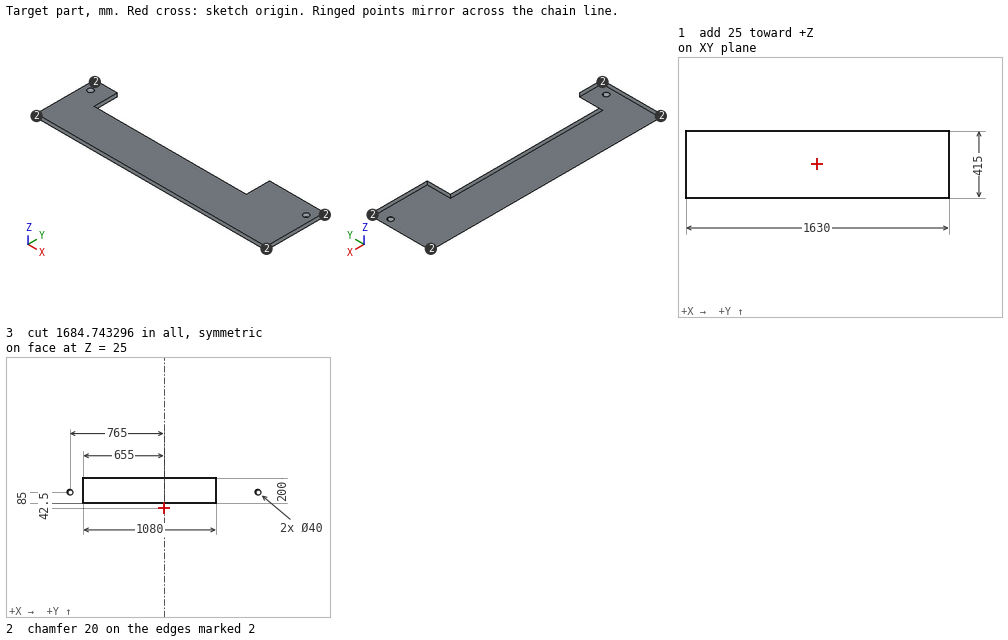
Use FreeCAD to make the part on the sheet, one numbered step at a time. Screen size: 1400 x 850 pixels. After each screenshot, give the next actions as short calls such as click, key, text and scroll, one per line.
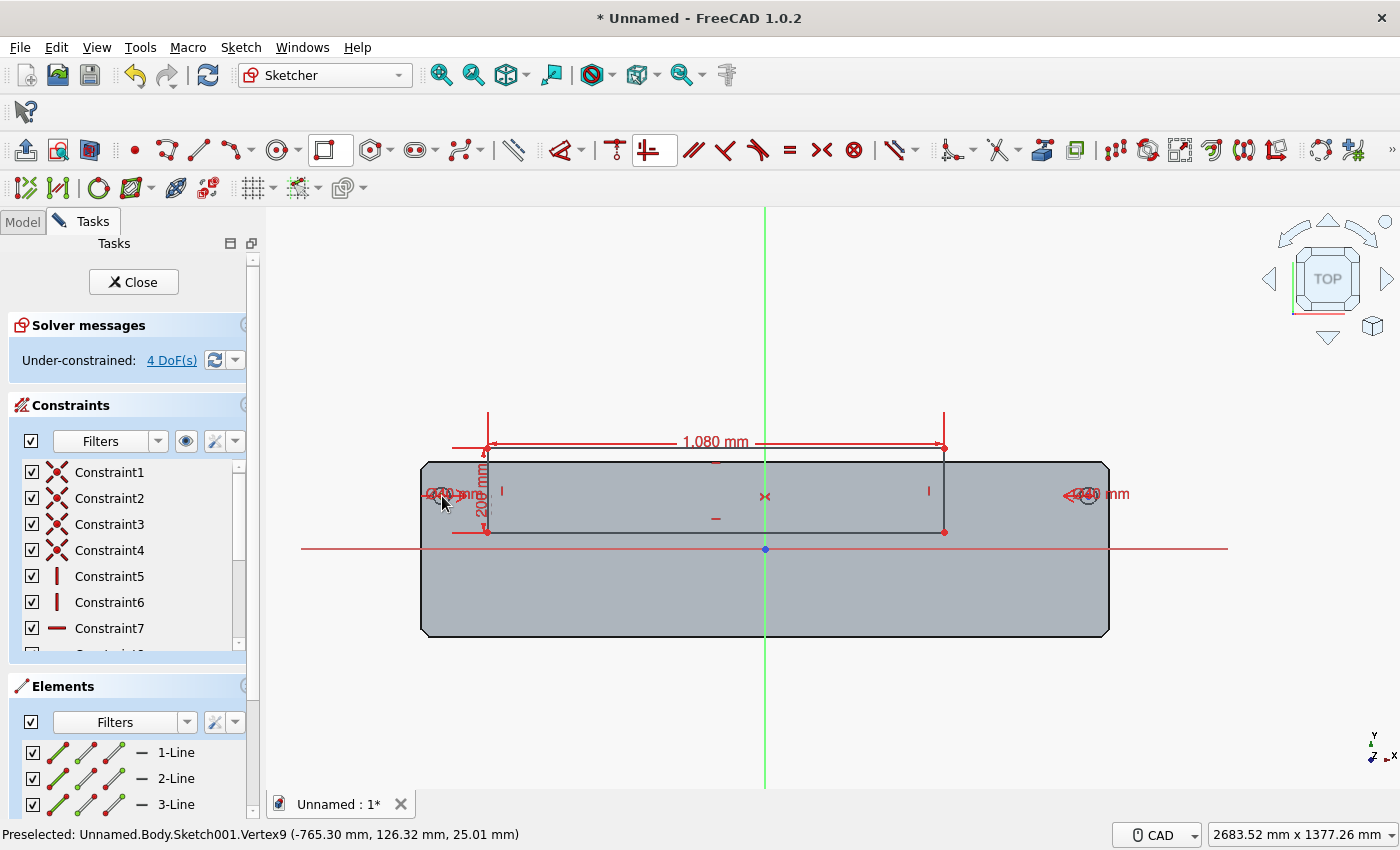
key(l)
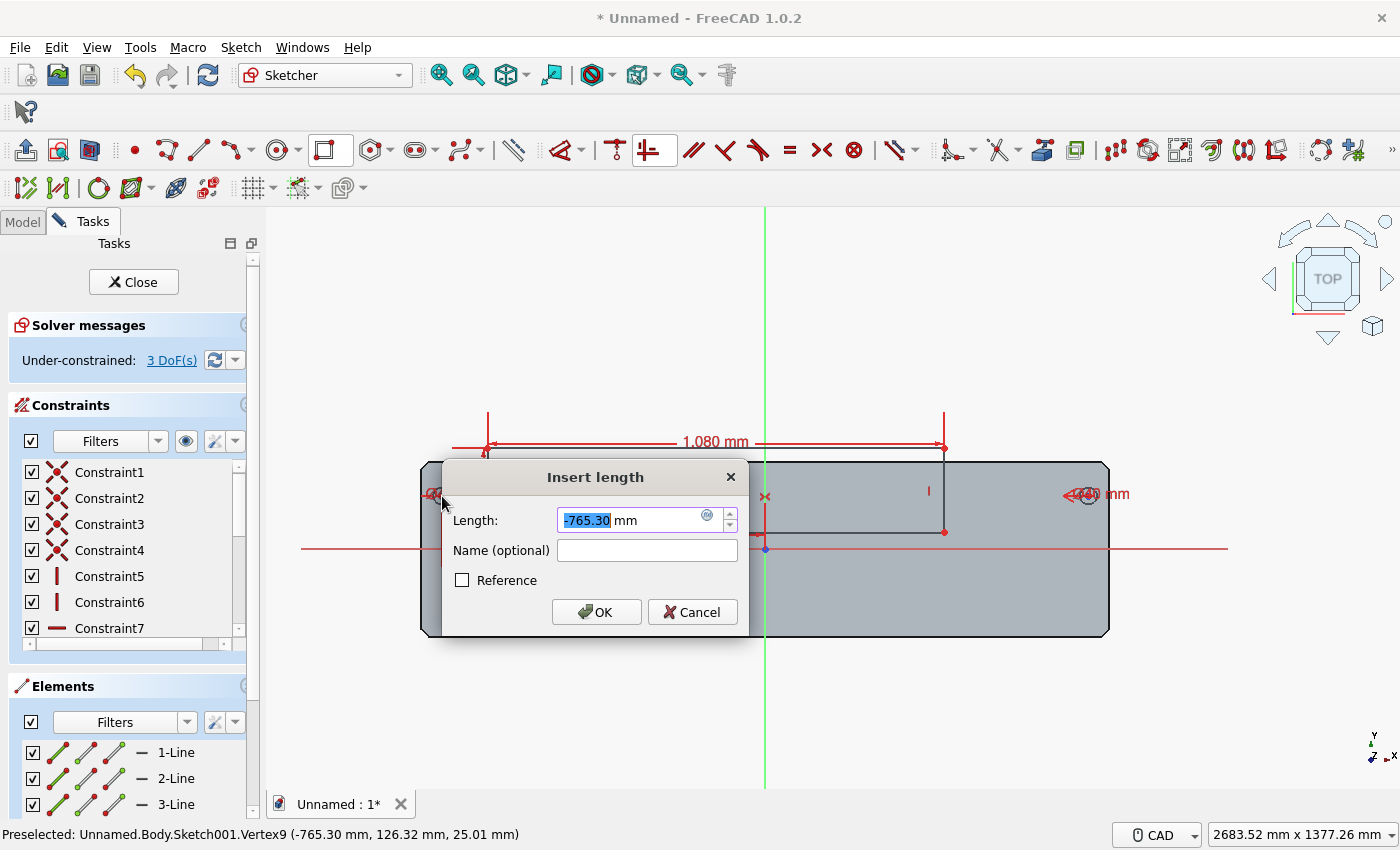
text(-765)
key(Return)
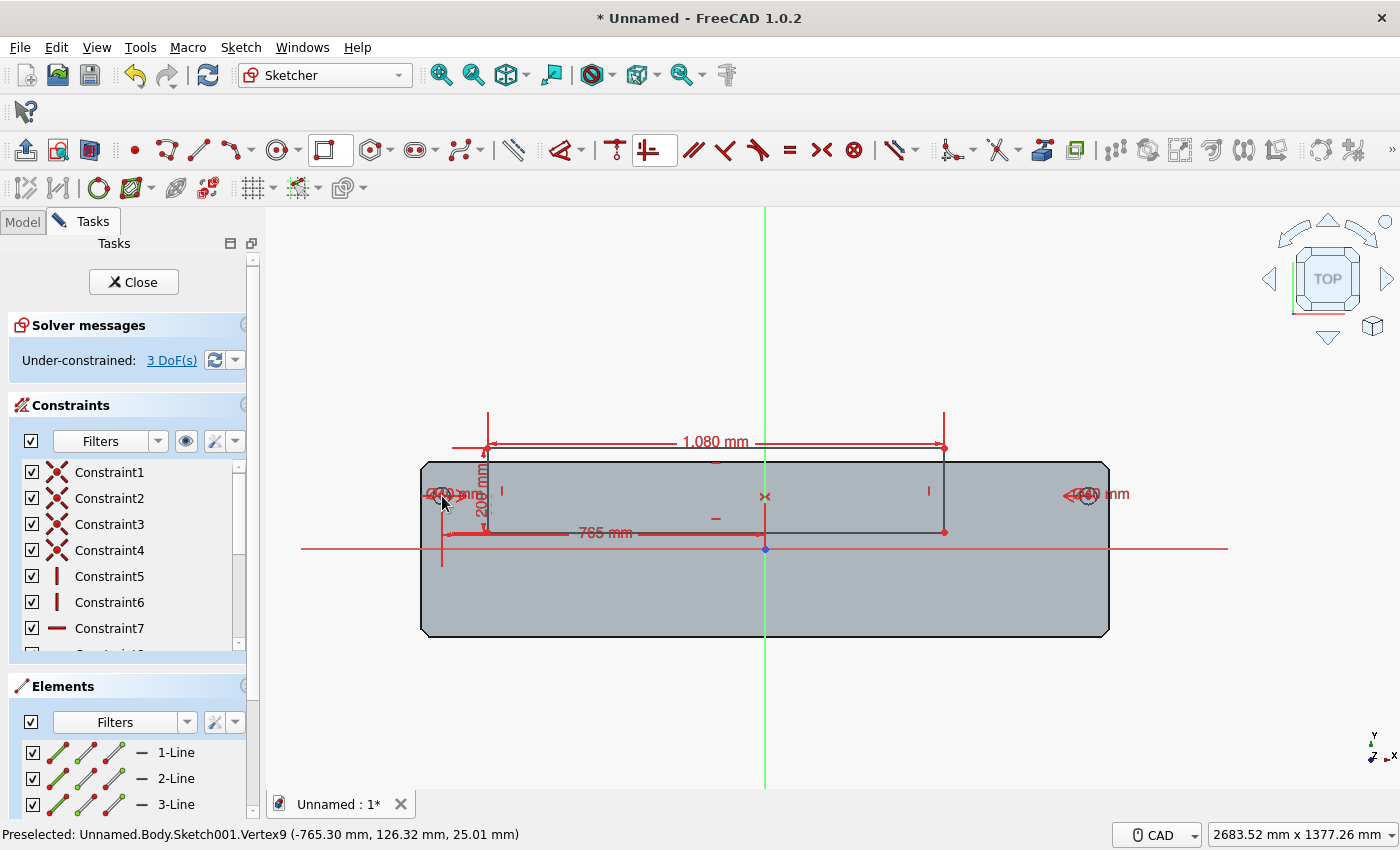
click(488, 533)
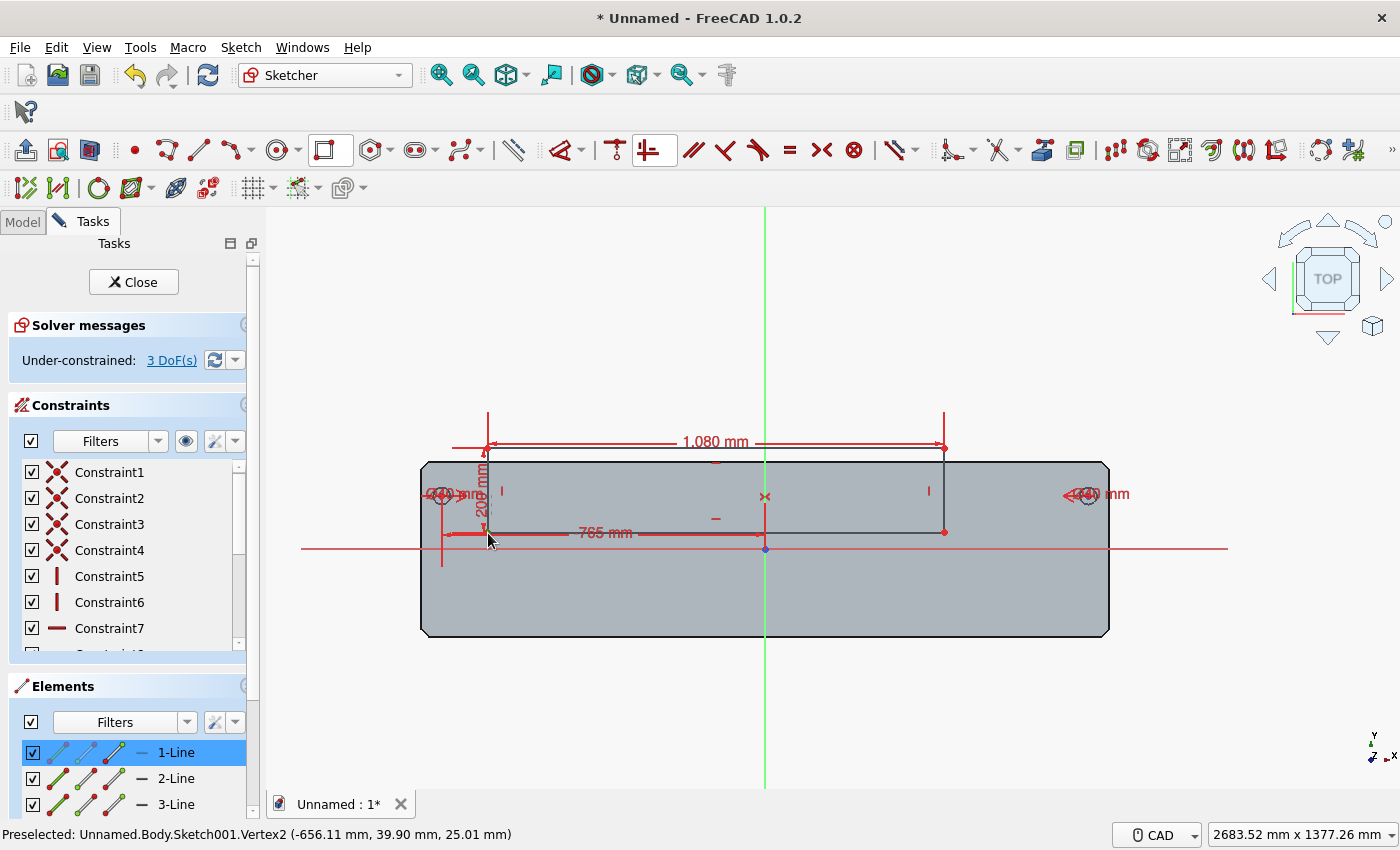
click(442, 496)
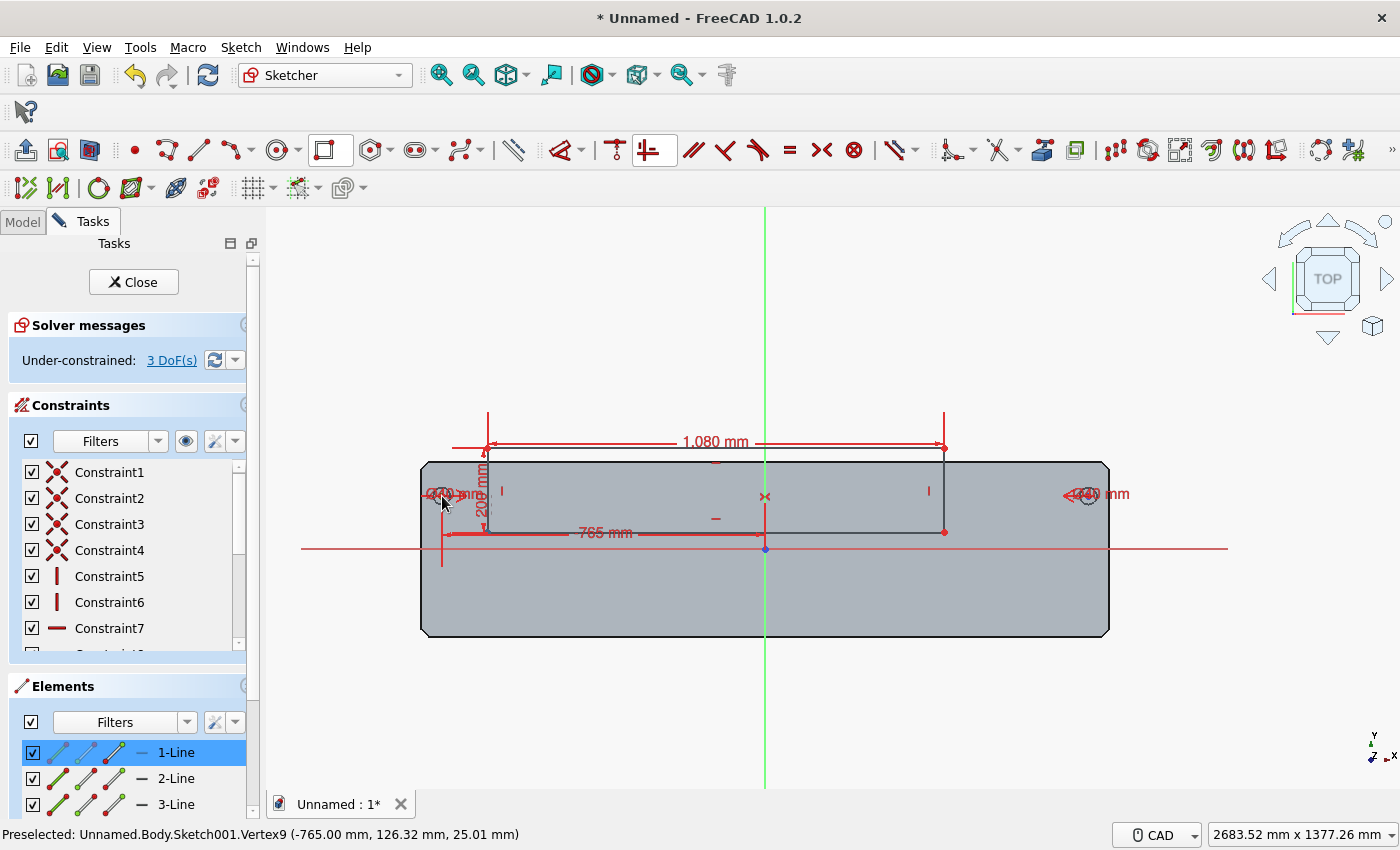
key(i)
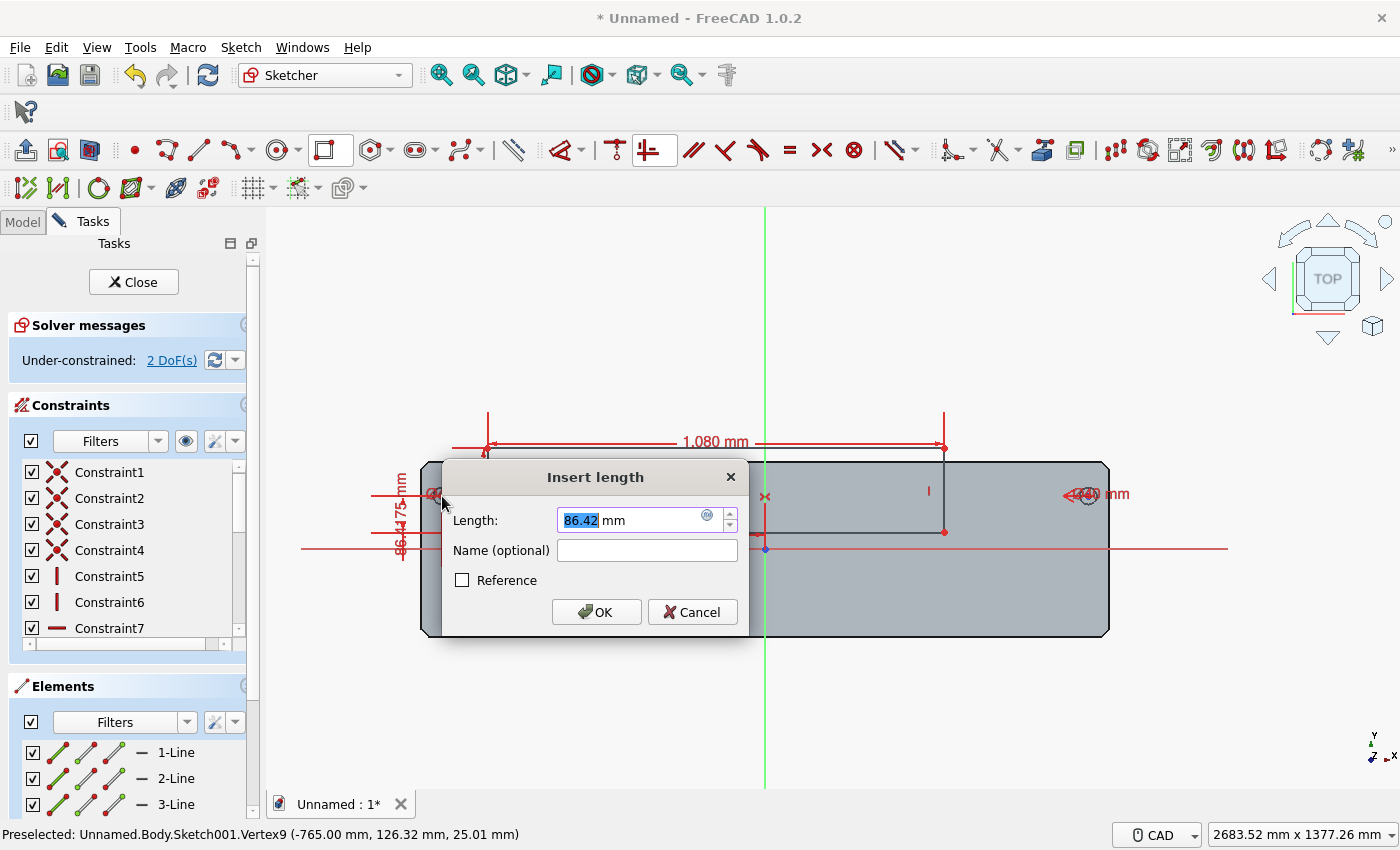
text(85)
key(Return)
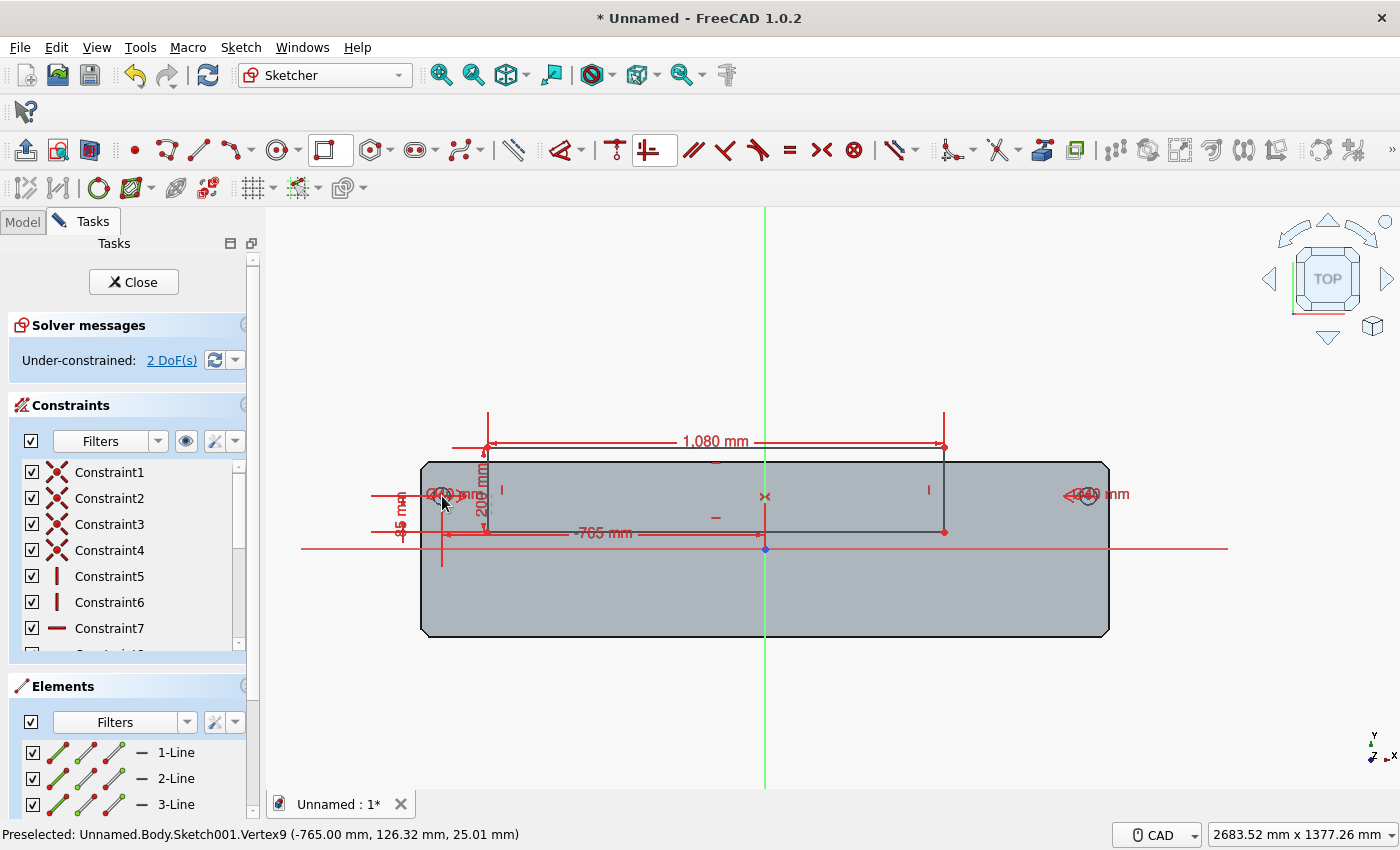
click(488, 448)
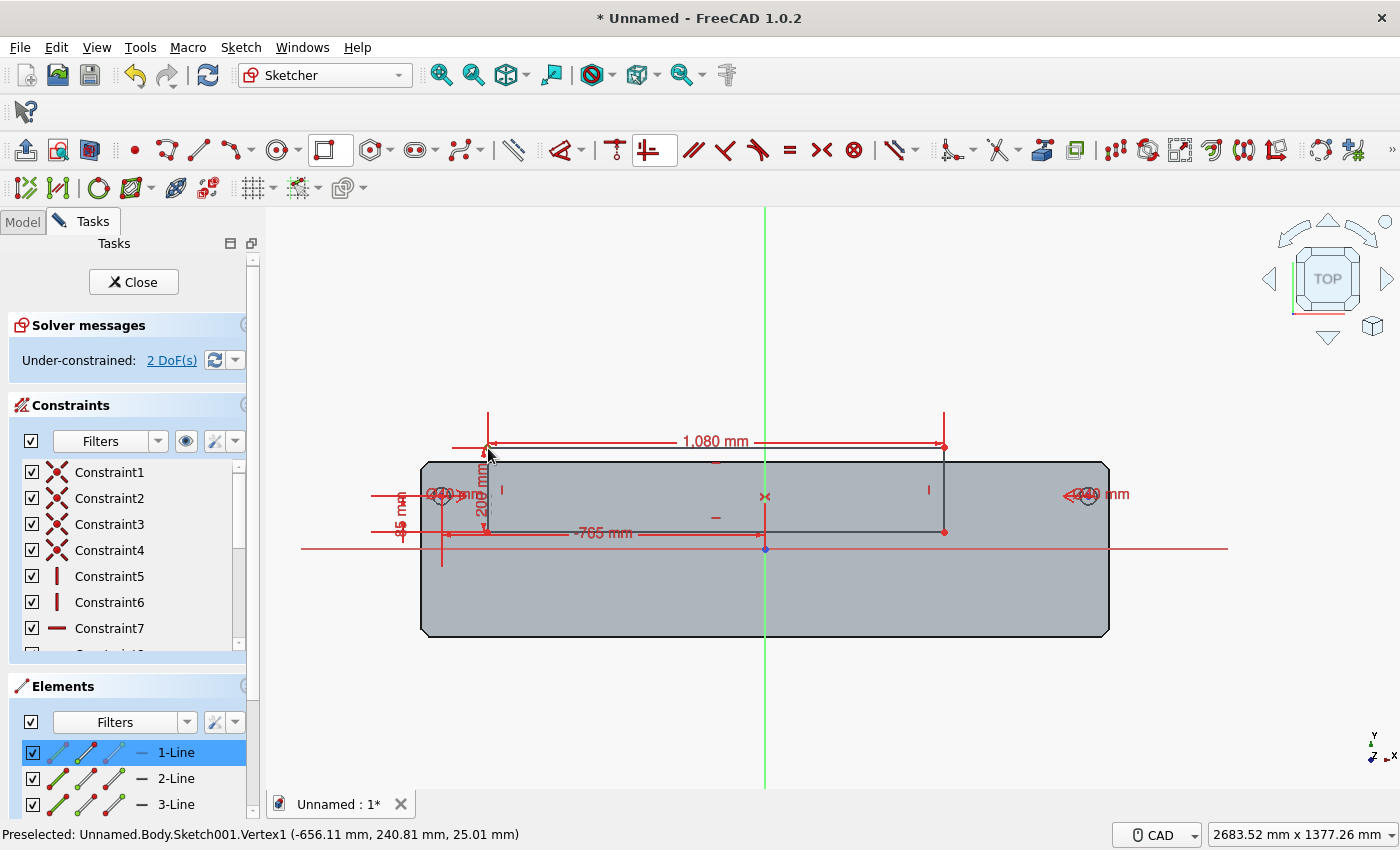
key(l)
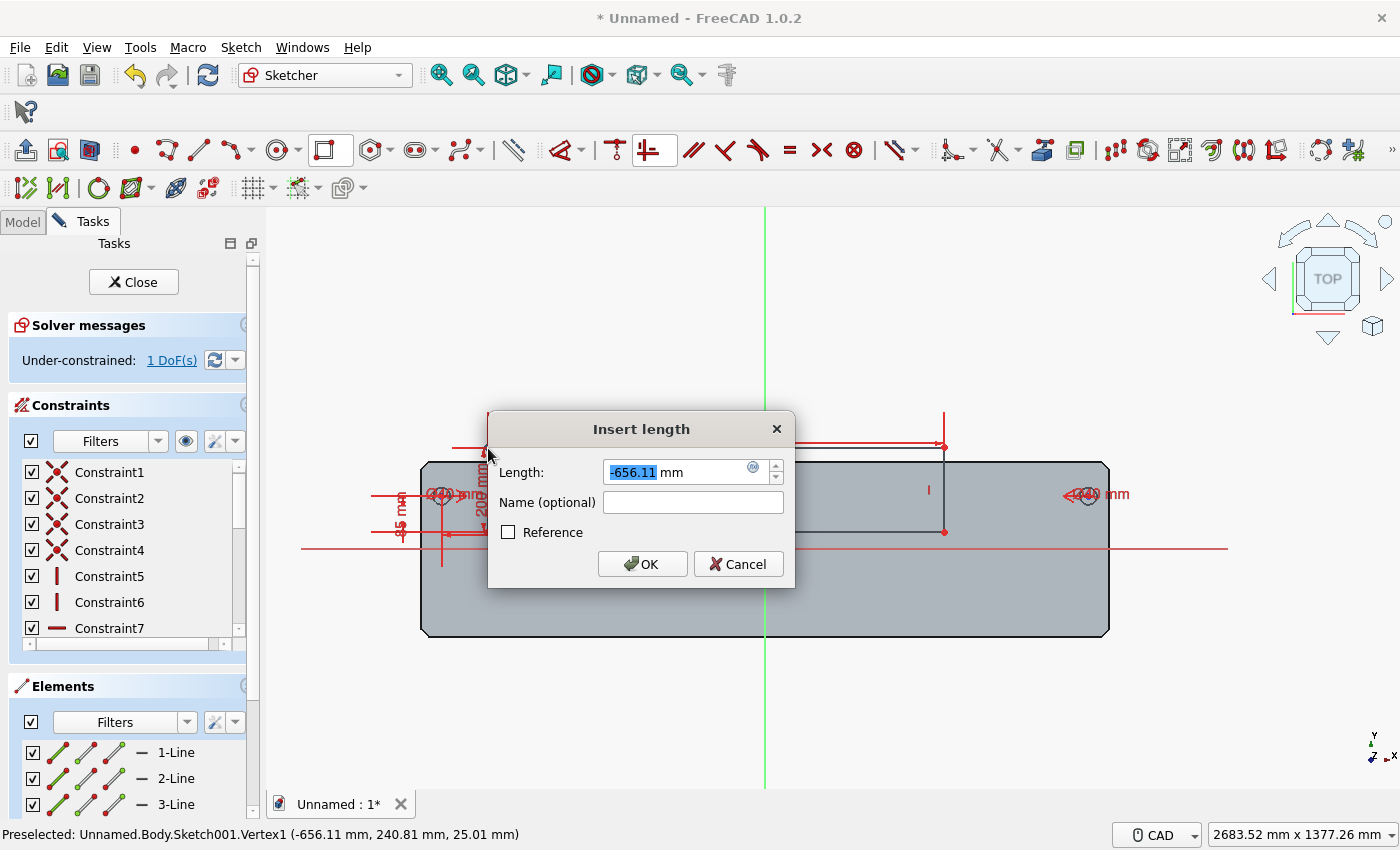
text(-655)
key(Return)